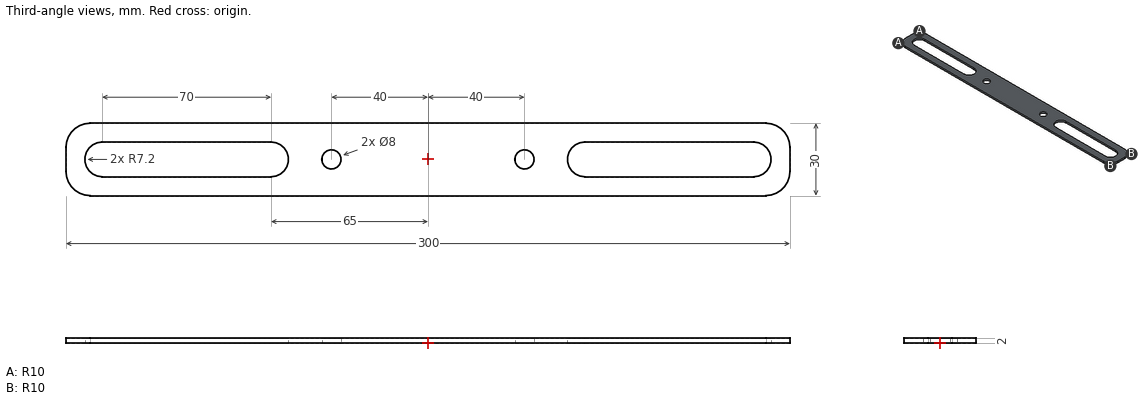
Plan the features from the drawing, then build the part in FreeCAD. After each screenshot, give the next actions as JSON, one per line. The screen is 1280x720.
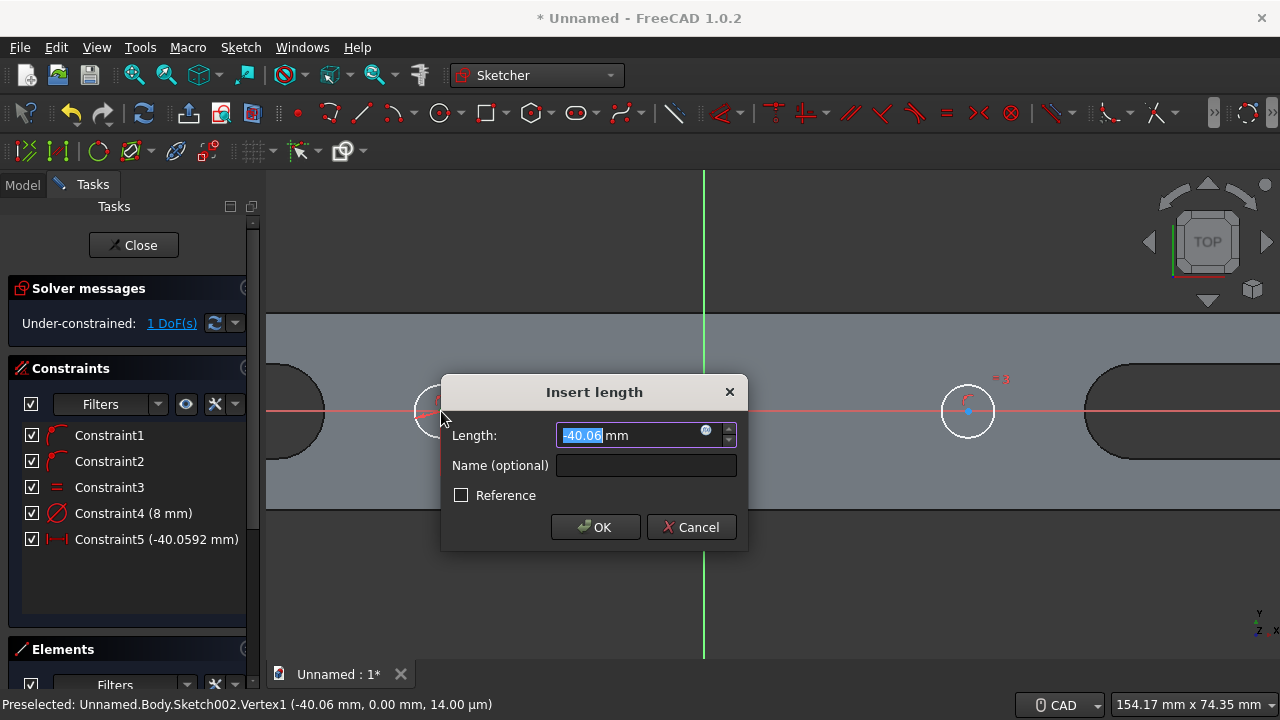
{"action": "type", "text": "-40"}
{"action": "key", "text": "Return"}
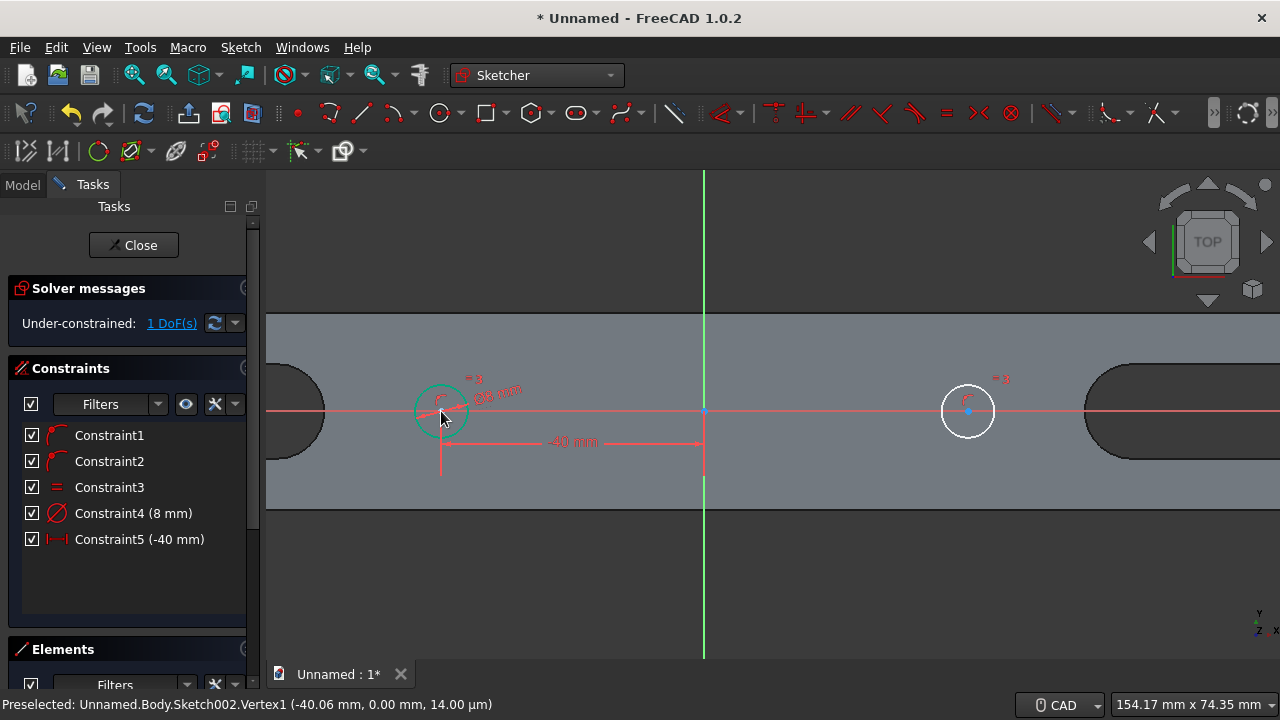
{"action": "left_click", "coordinate": [968, 411]}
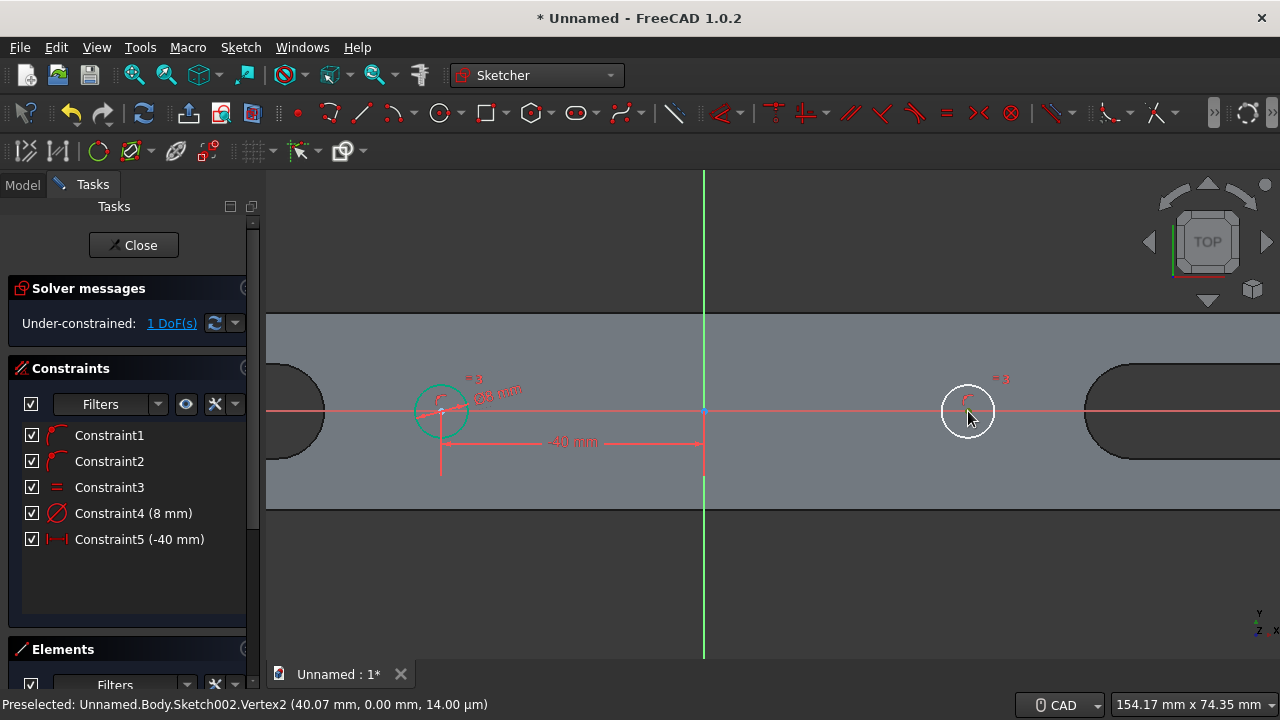
{"action": "key", "text": "l"}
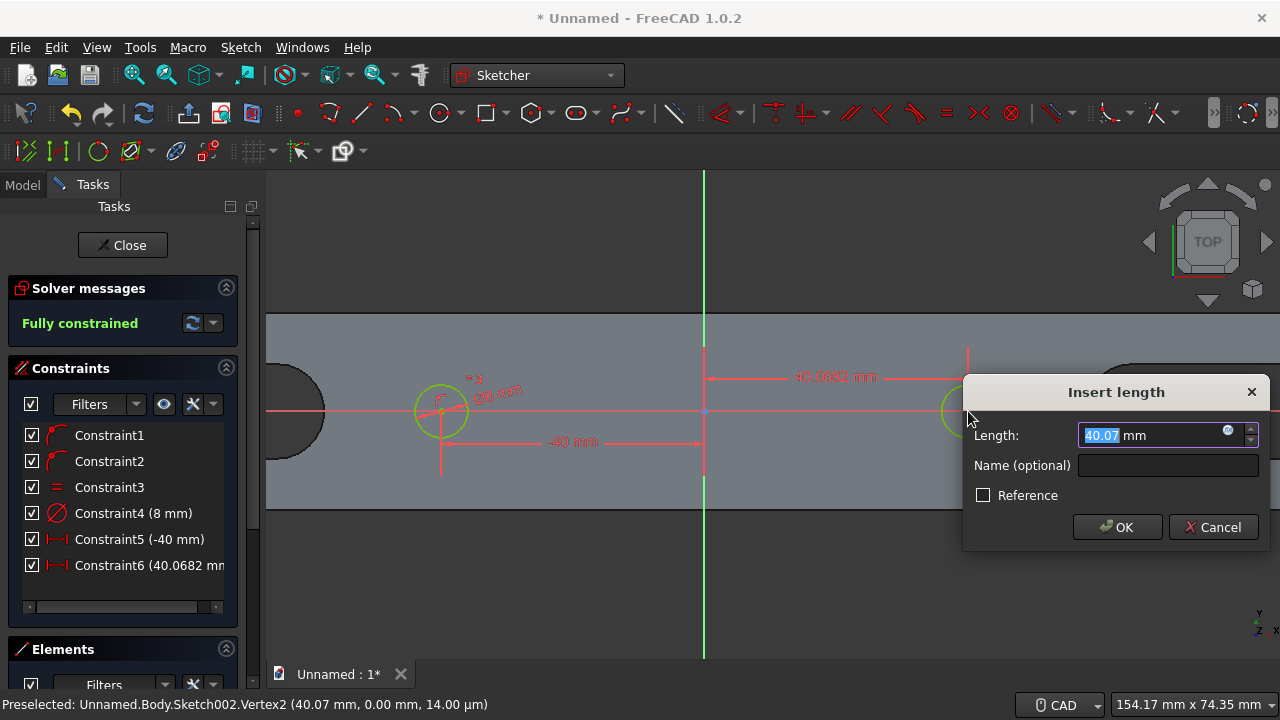
{"action": "type", "text": "40"}
{"action": "key", "text": "Return"}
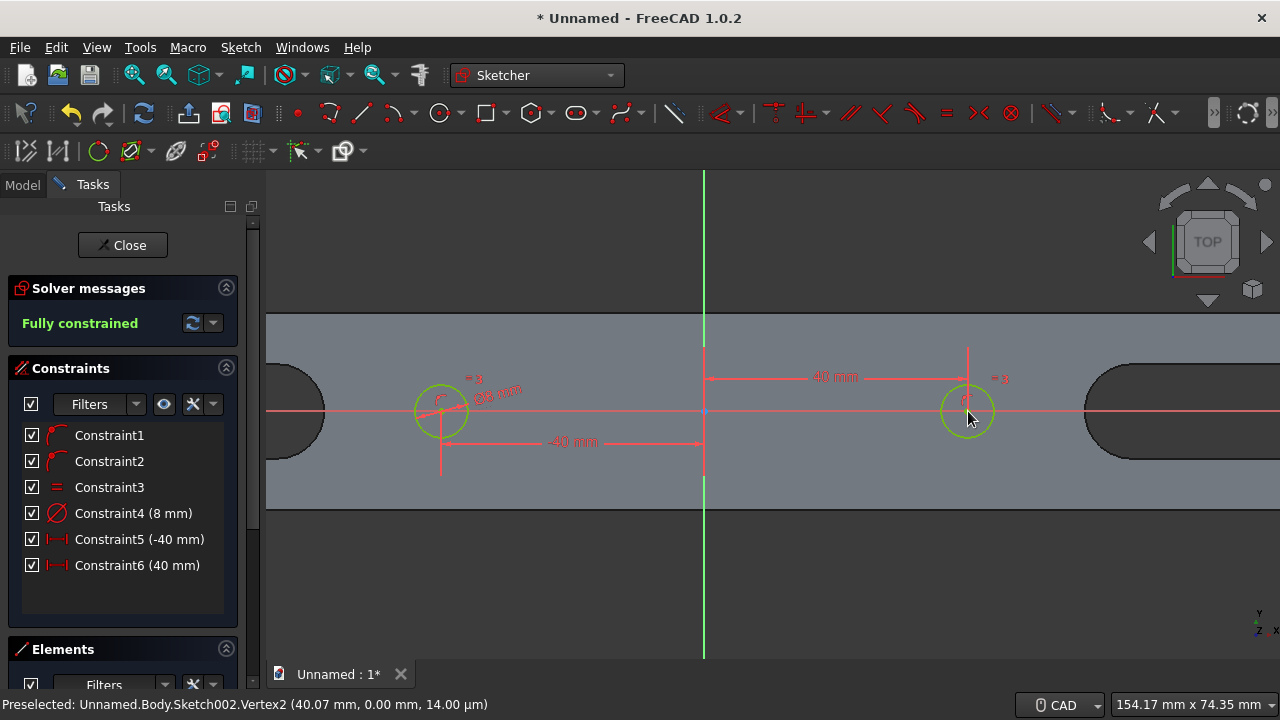
{"action": "left_click", "coordinate": [123, 245]}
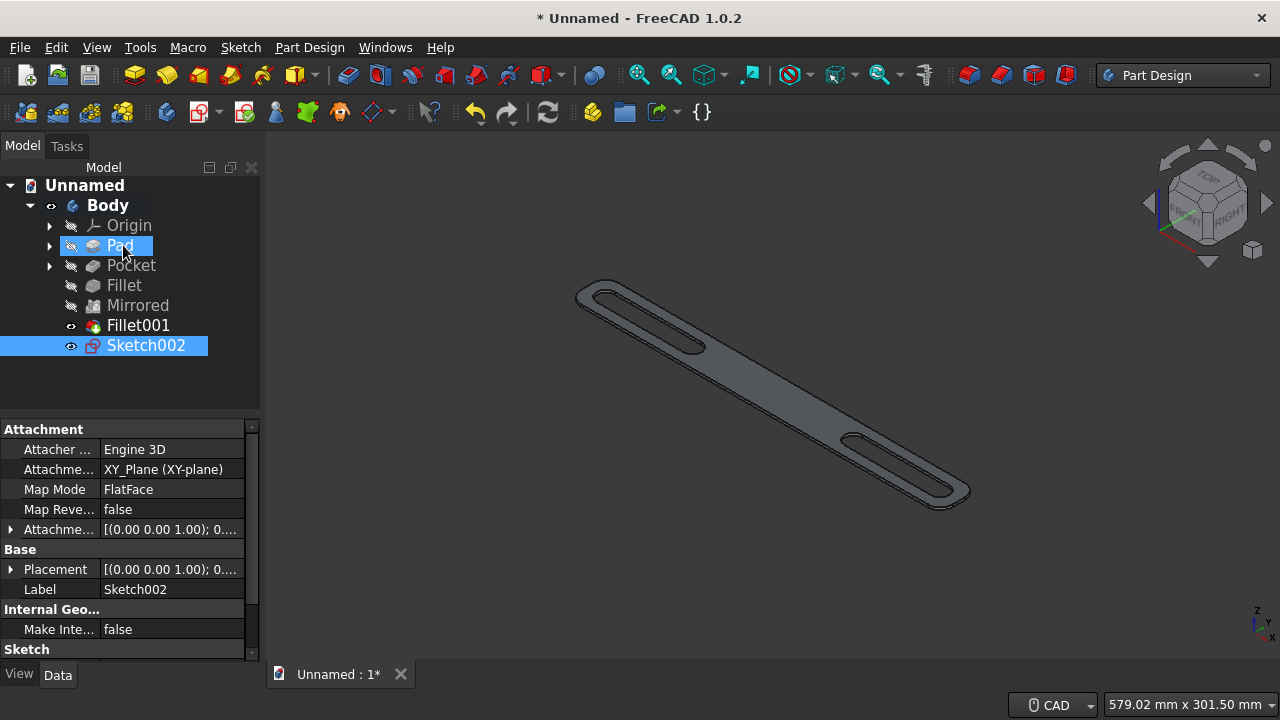
{"action": "left_click", "coordinate": [350, 76]}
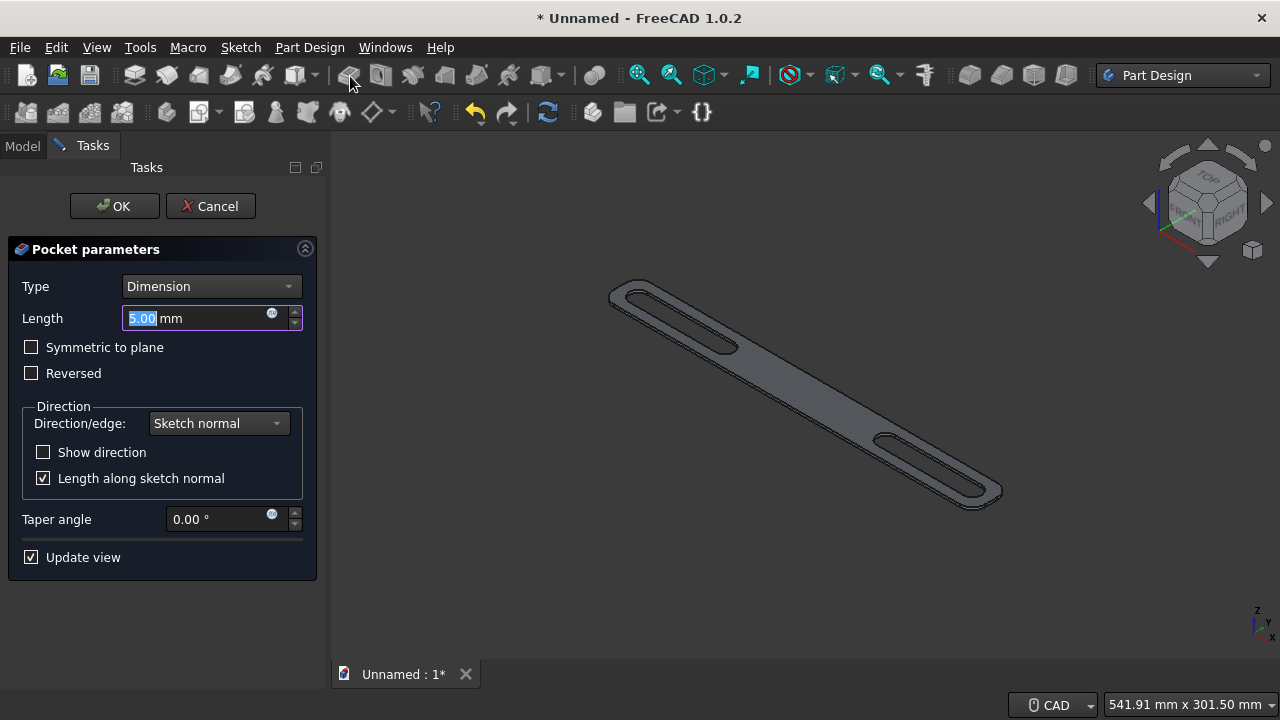
{"action": "left_click", "coordinate": [212, 286]}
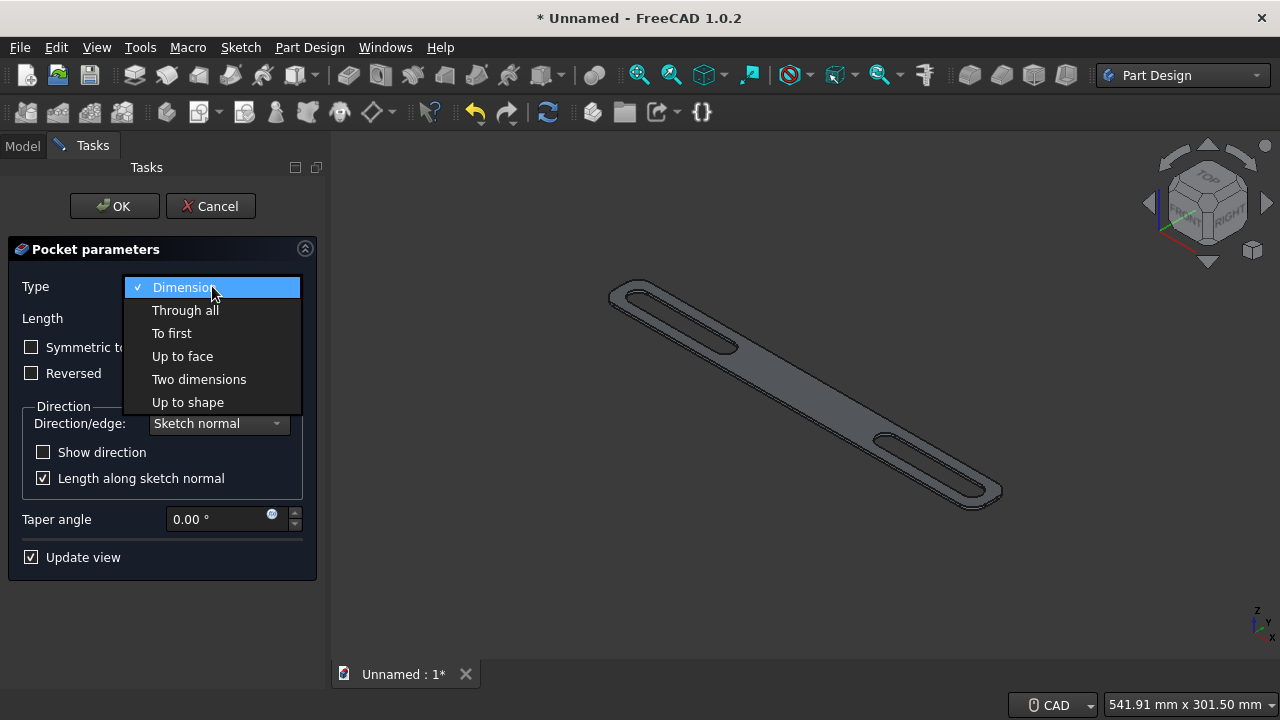
{"action": "left_click", "coordinate": [212, 310]}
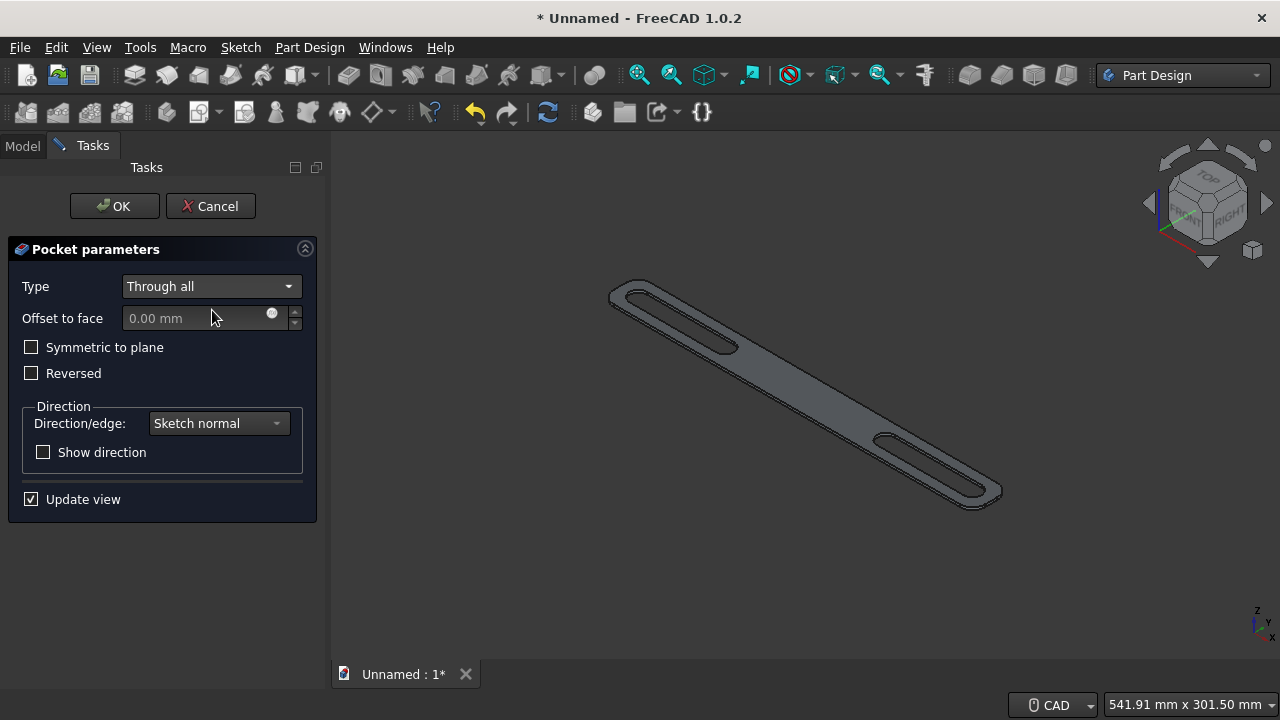
{"action": "left_click", "coordinate": [30, 373]}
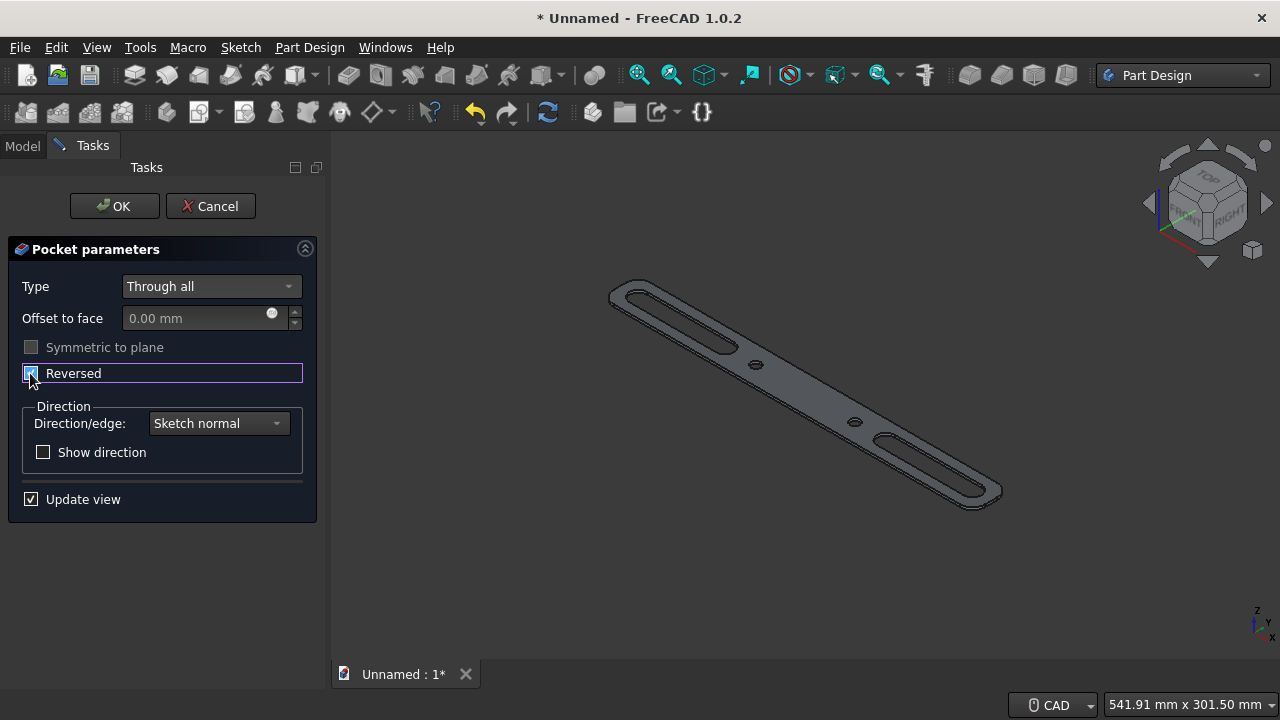
{"action": "left_click", "coordinate": [115, 206]}